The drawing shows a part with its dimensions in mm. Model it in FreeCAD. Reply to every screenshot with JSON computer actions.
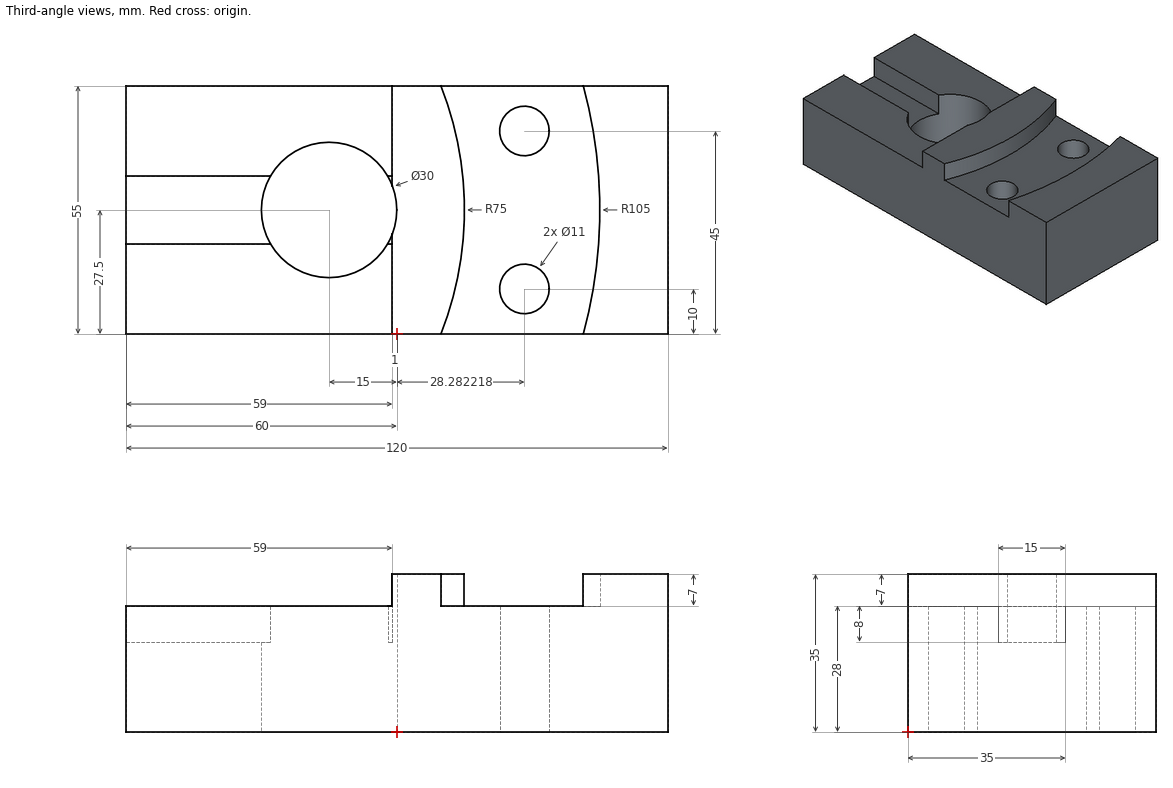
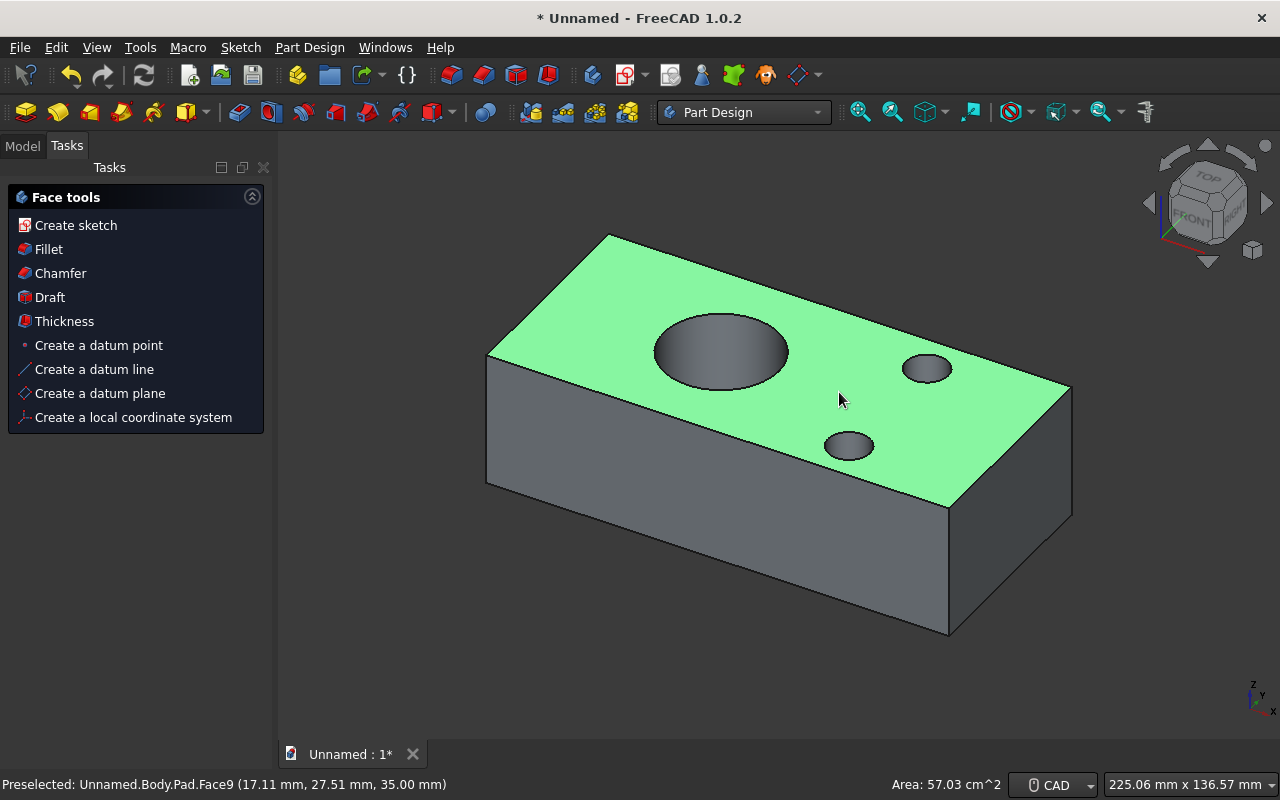
{"action": "left_click", "coordinate": [626, 76]}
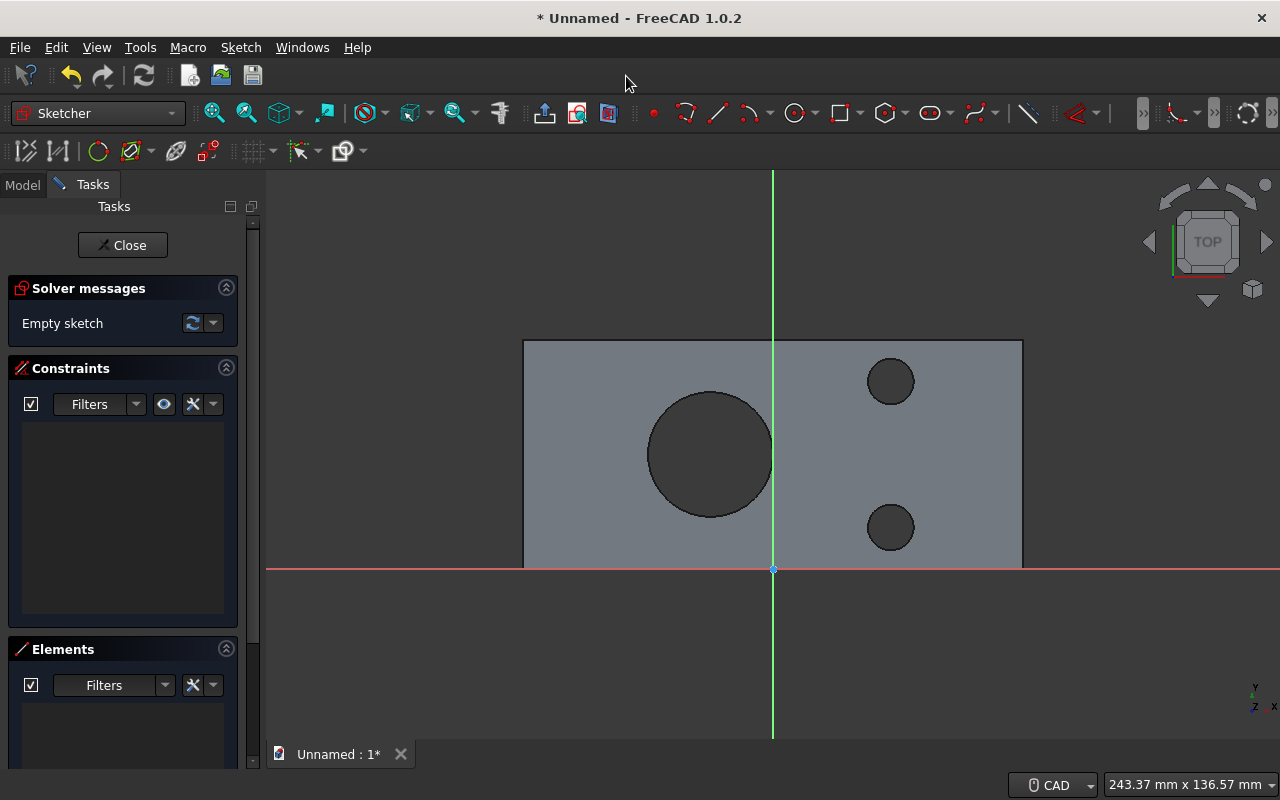
{"action": "scroll", "coordinate": [1115, 455], "scroll_direction": "up", "scroll_amount": 2}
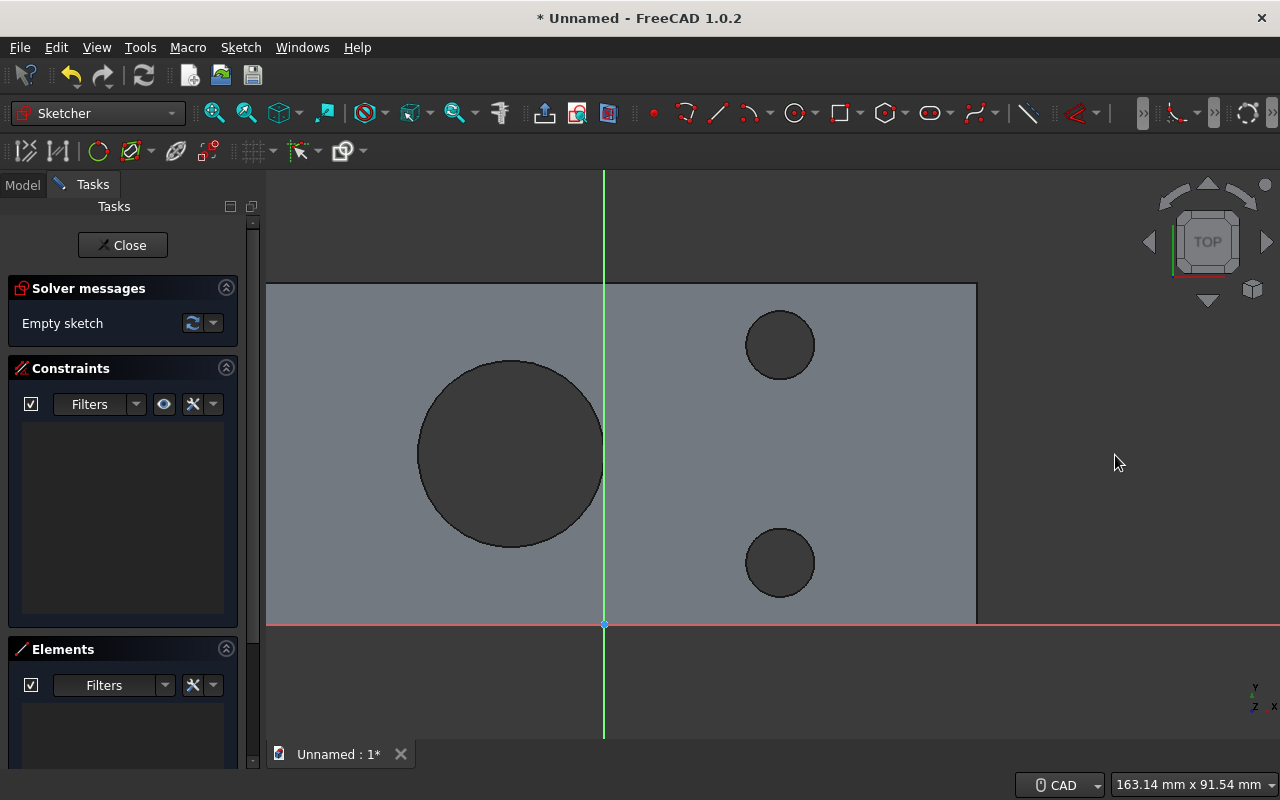
{"action": "left_click", "coordinate": [718, 114]}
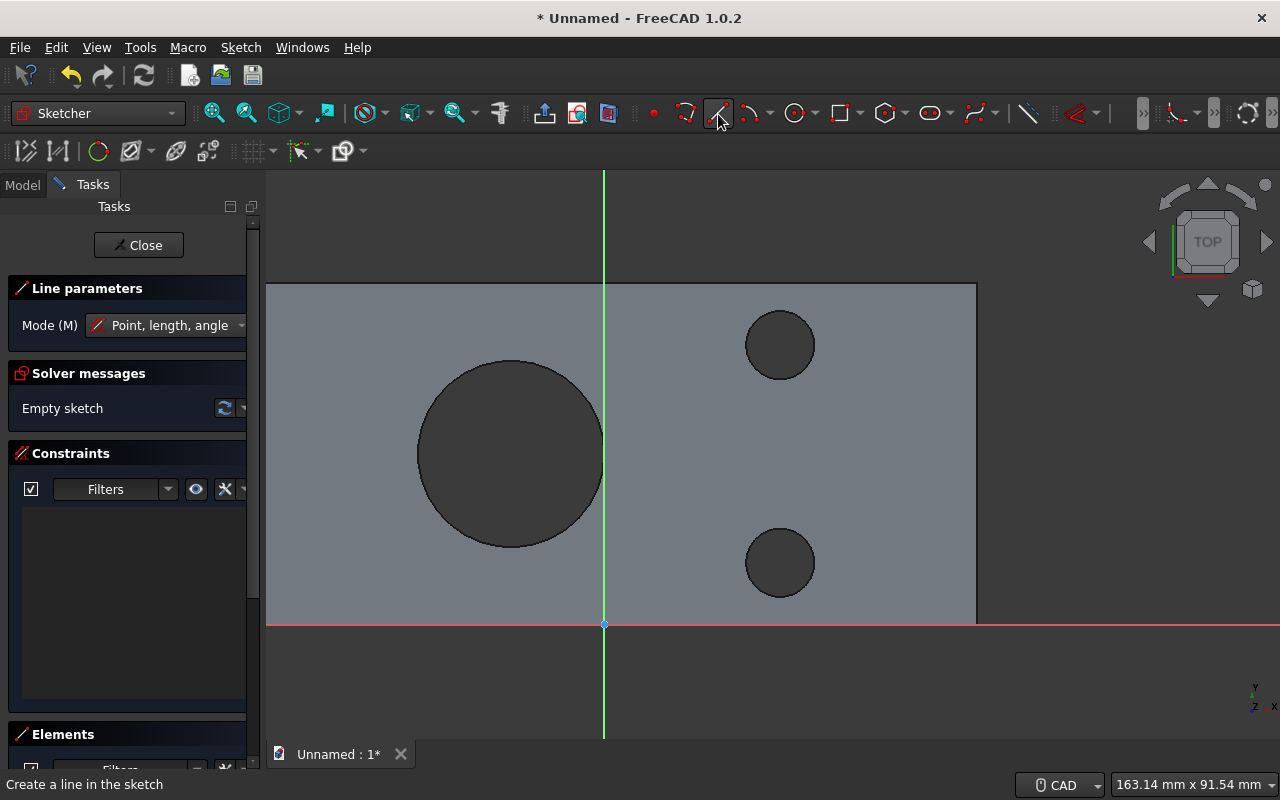
{"action": "left_click", "coordinate": [861, 283]}
{"action": "left_click", "coordinate": [665, 283]}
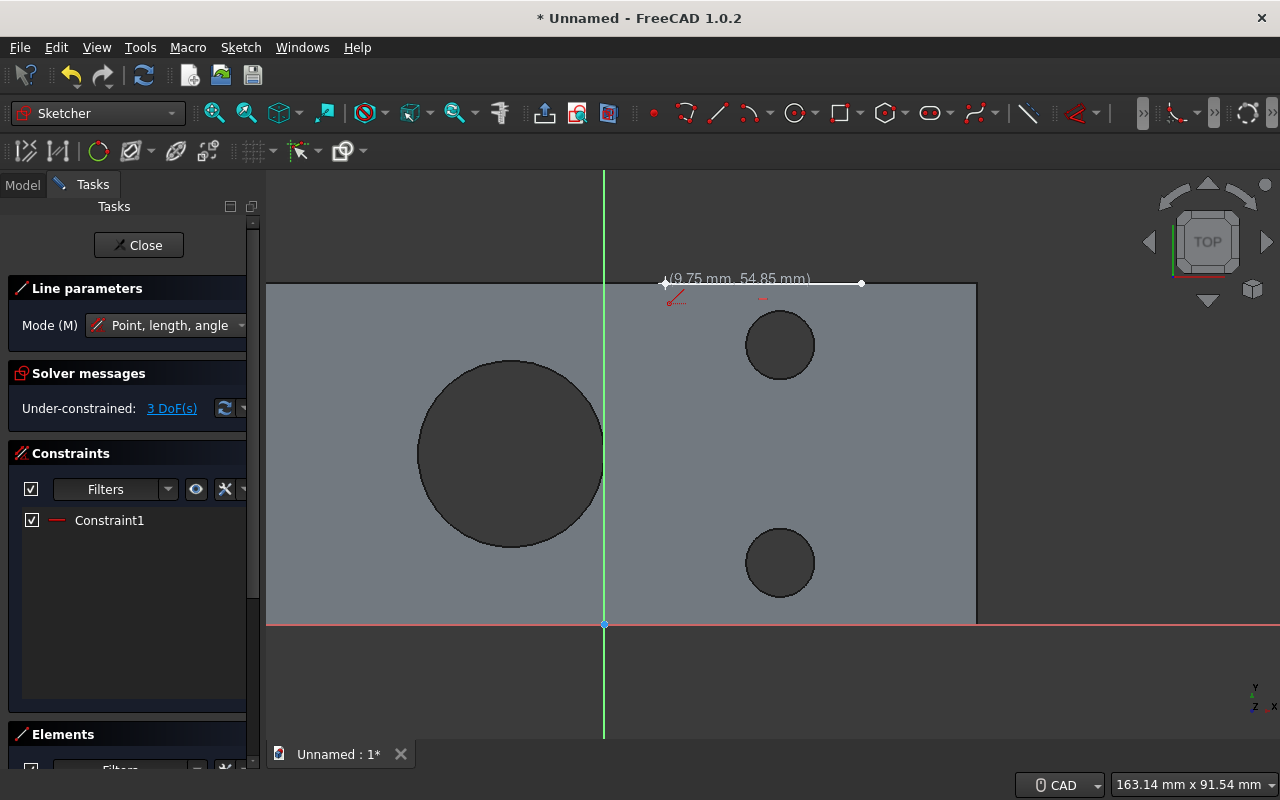
{"action": "left_click", "coordinate": [665, 625]}
{"action": "left_click", "coordinate": [861, 616]}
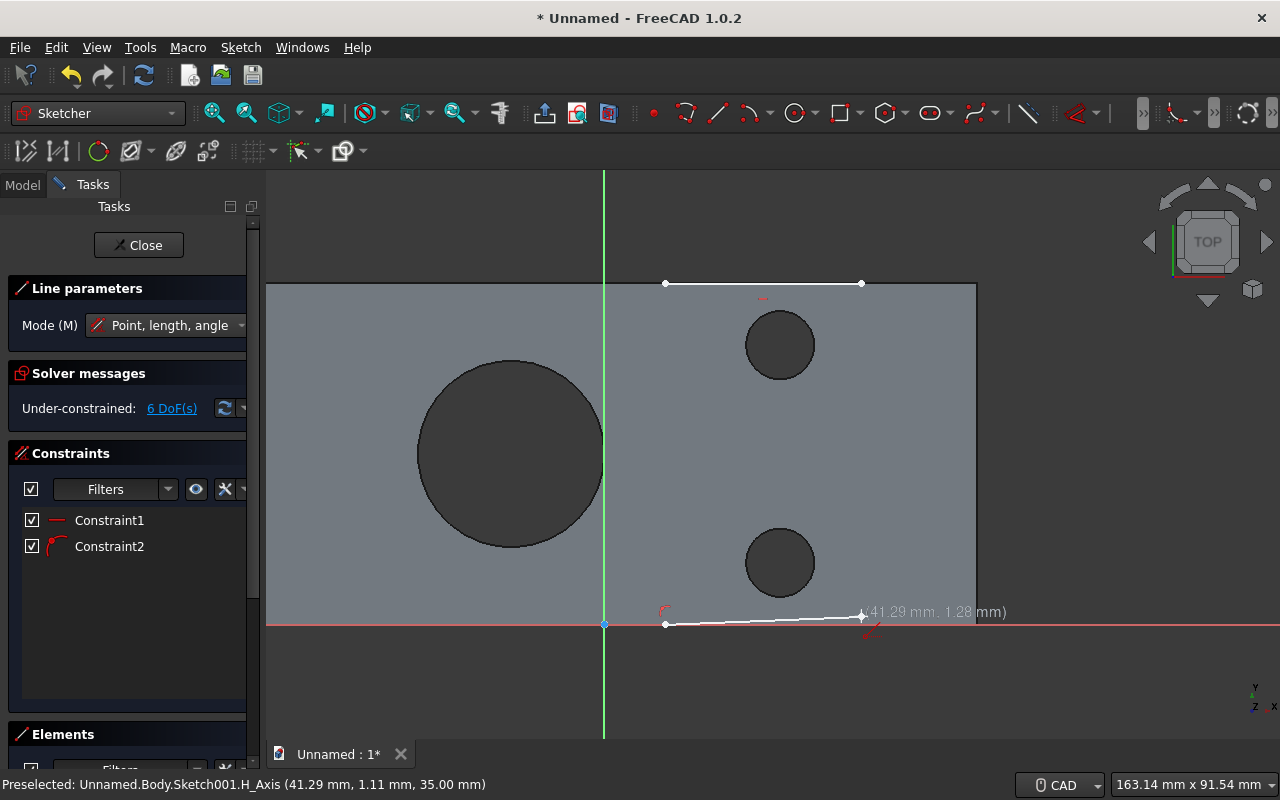
{"action": "key", "text": "g 3 a"}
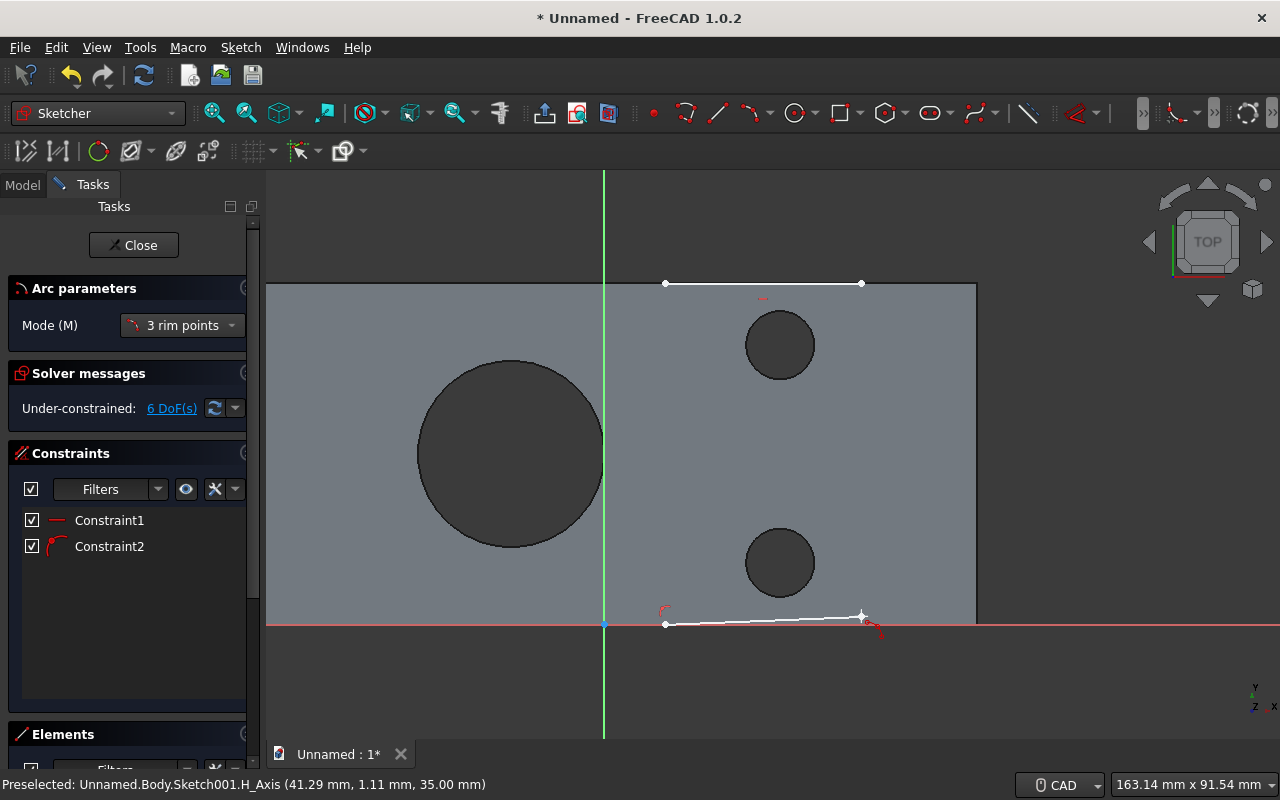
{"action": "left_click", "coordinate": [665, 284]}
{"action": "left_click", "coordinate": [665, 625]}
{"action": "left_click", "coordinate": [698, 454]}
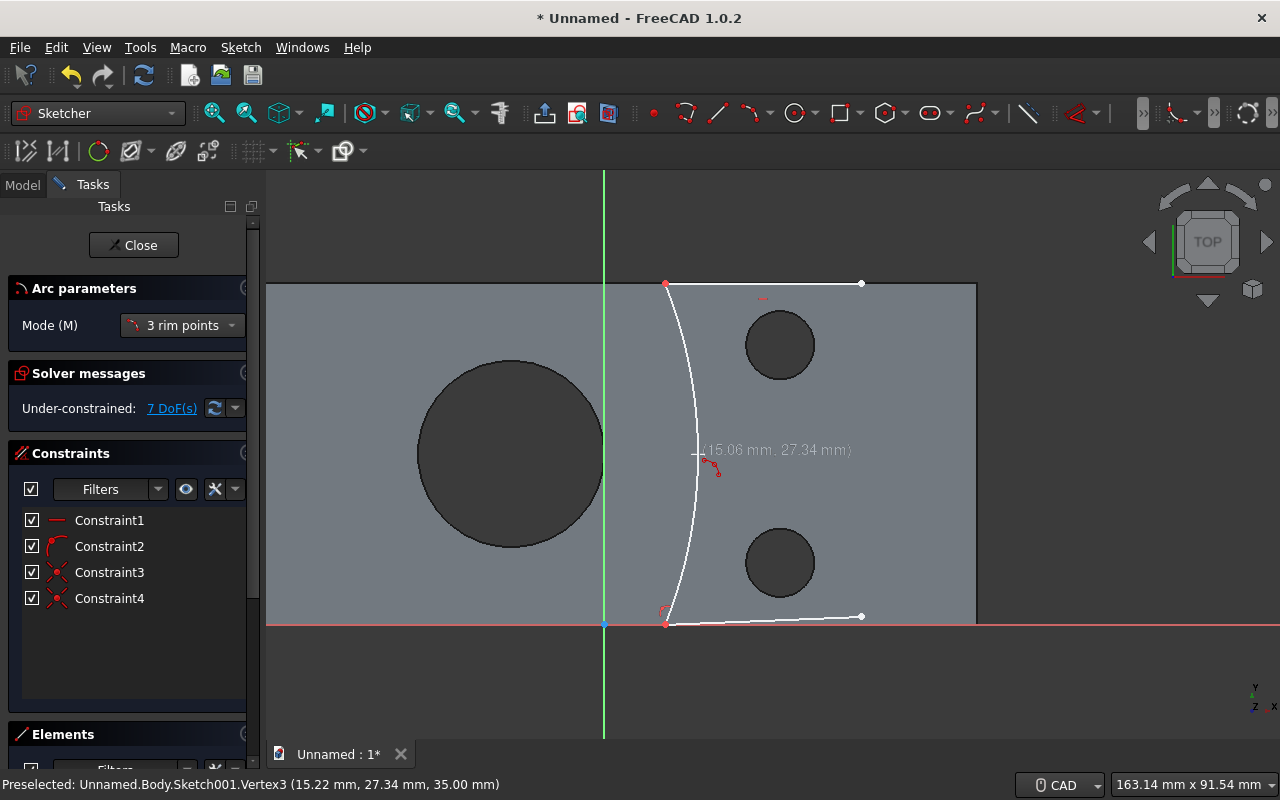
{"action": "left_click", "coordinate": [861, 617]}
{"action": "left_click", "coordinate": [861, 284]}
{"action": "left_click", "coordinate": [884, 454]}
{"action": "key", "text": "Escape"}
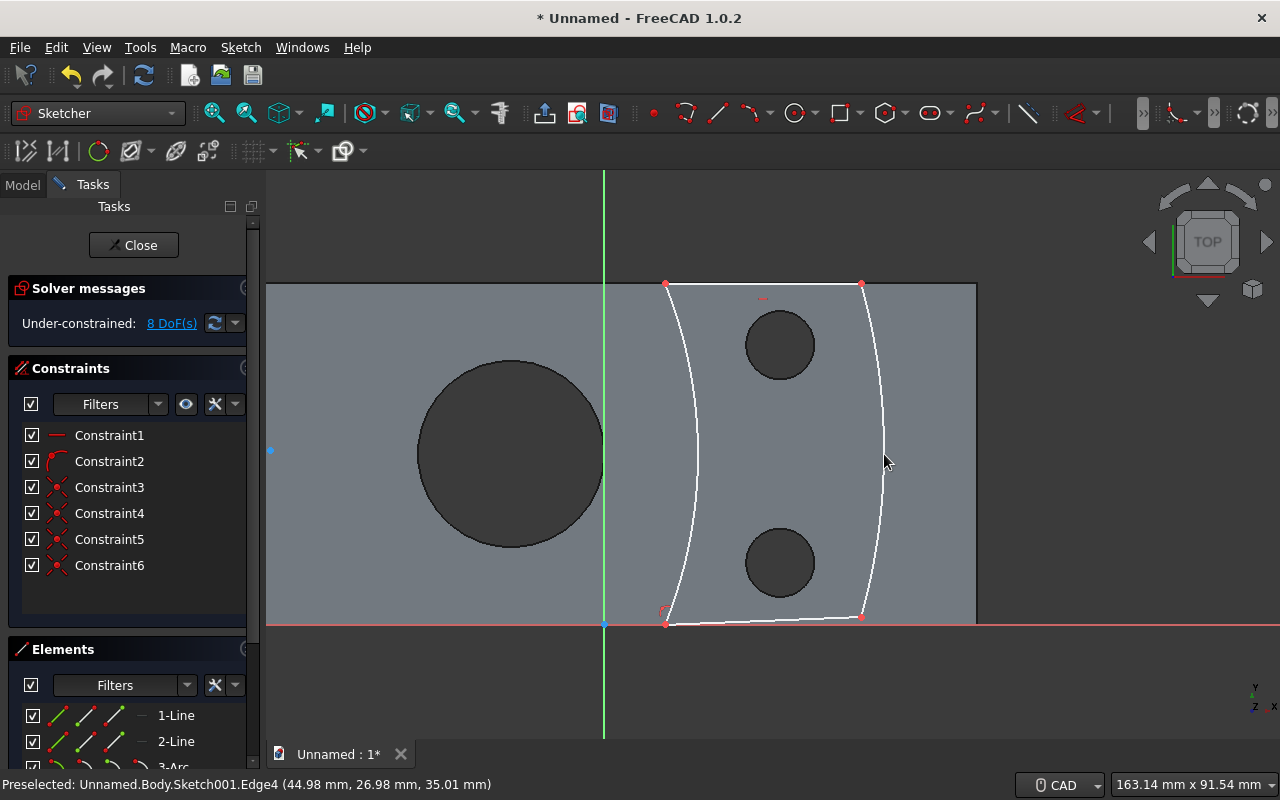
{"action": "left_click", "coordinate": [724, 623]}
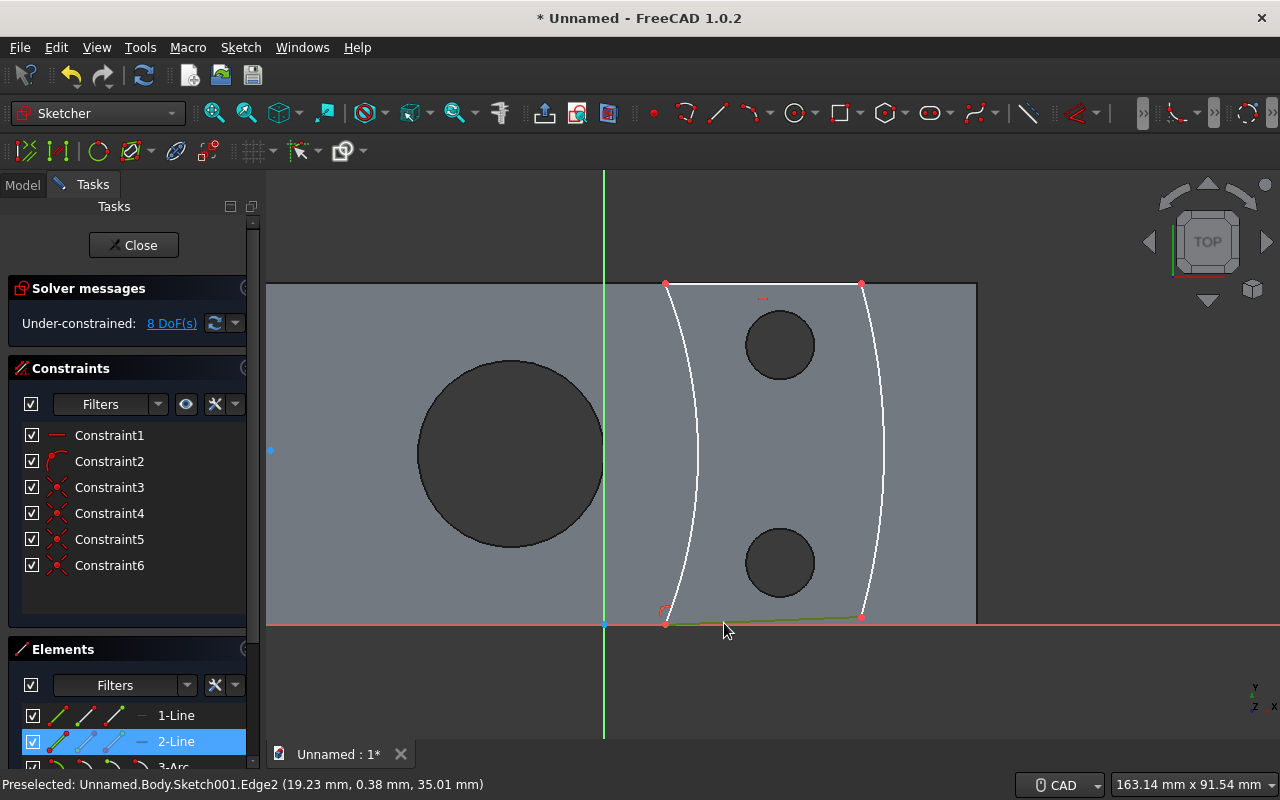
{"action": "key", "text": "h"}